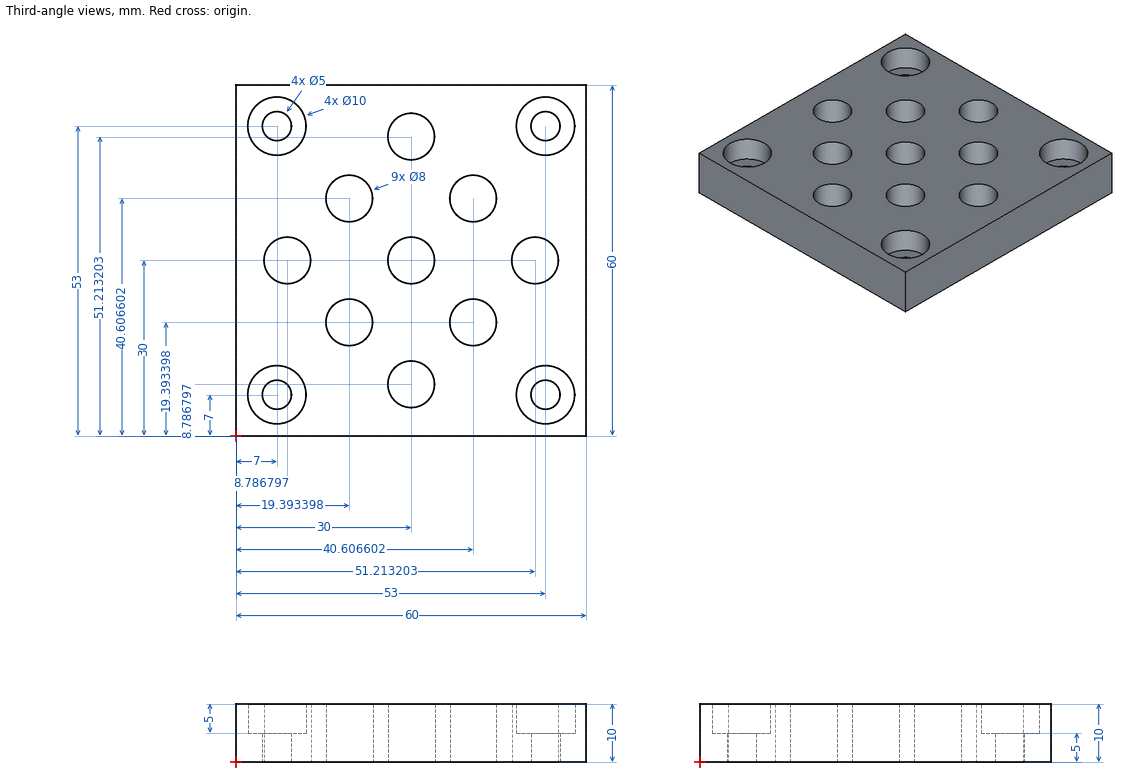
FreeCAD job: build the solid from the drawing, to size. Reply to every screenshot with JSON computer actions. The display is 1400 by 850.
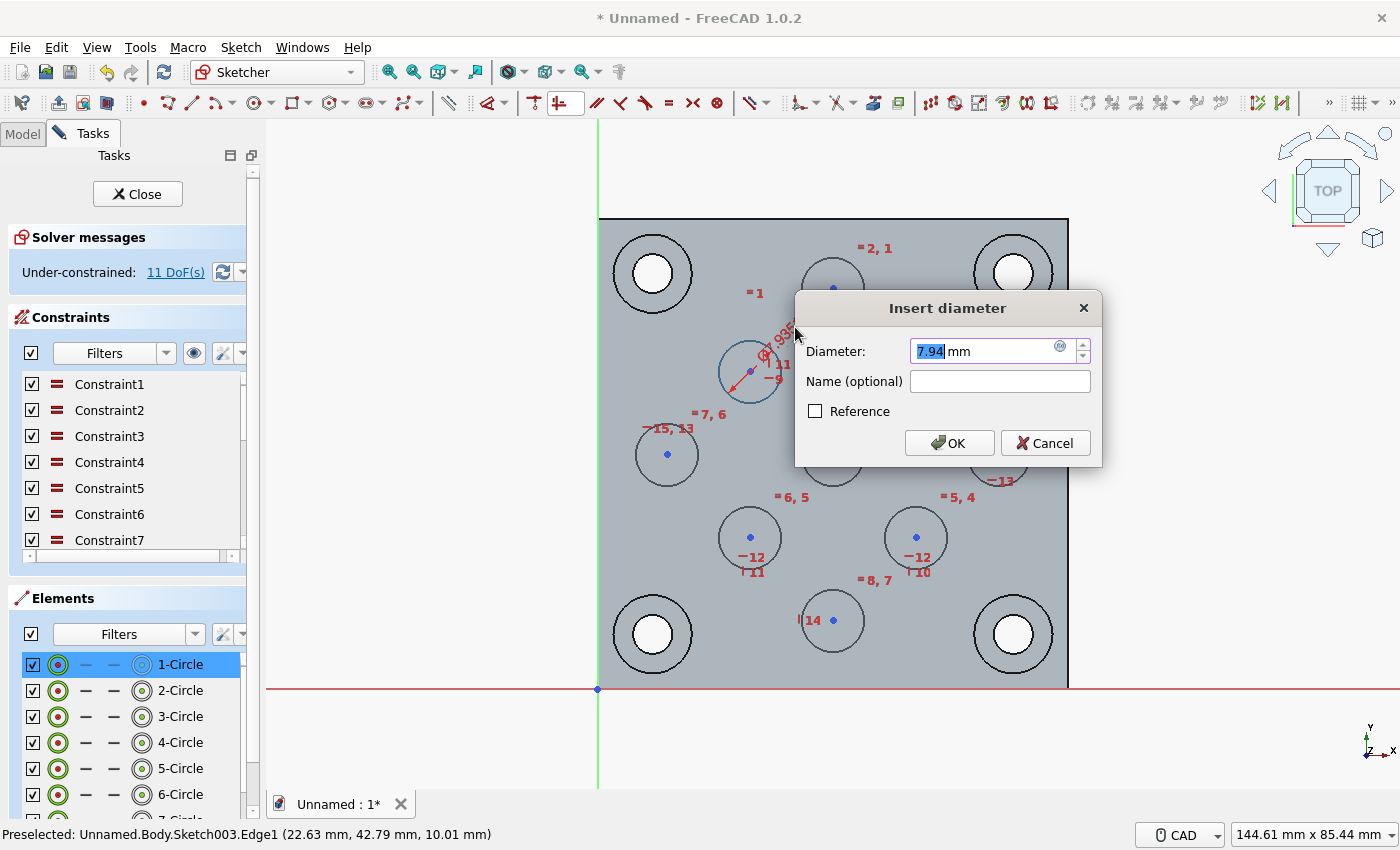
{"action": "type", "text": "8"}
{"action": "key", "text": "Return"}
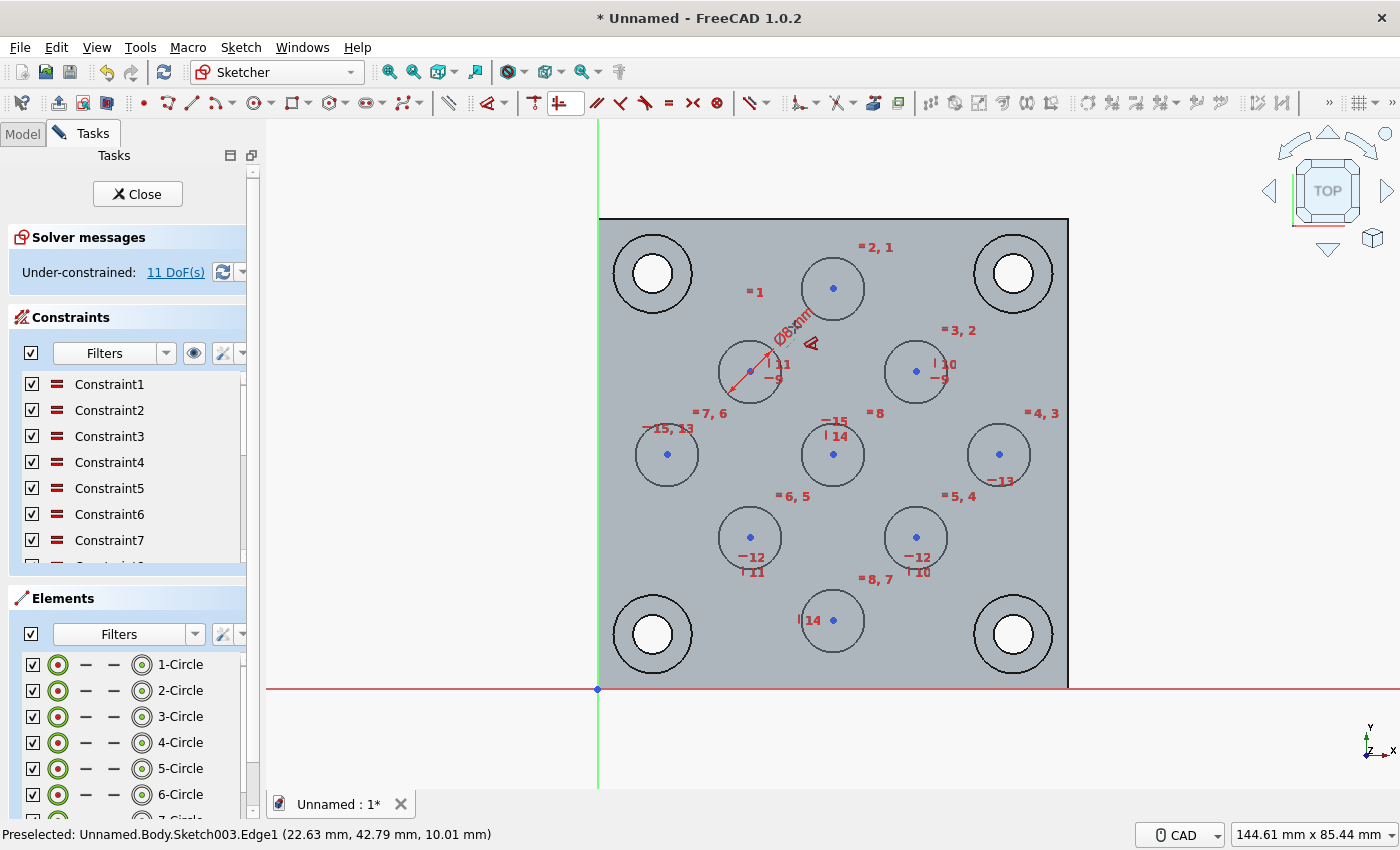
{"action": "left_click", "coordinate": [833, 289]}
{"action": "left_click", "coordinate": [715, 723]}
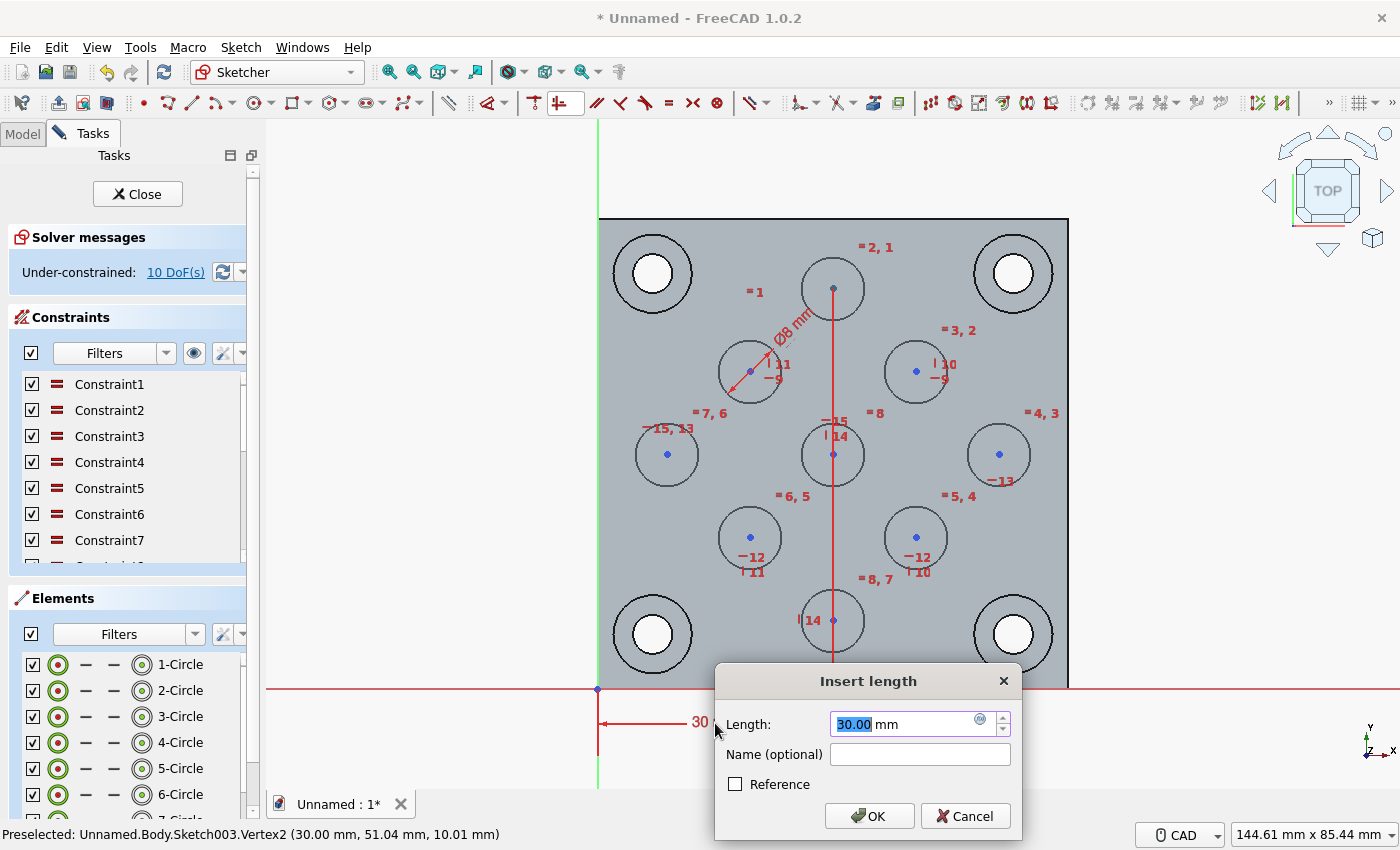
{"action": "type", "text": "30"}
{"action": "key", "text": "Return"}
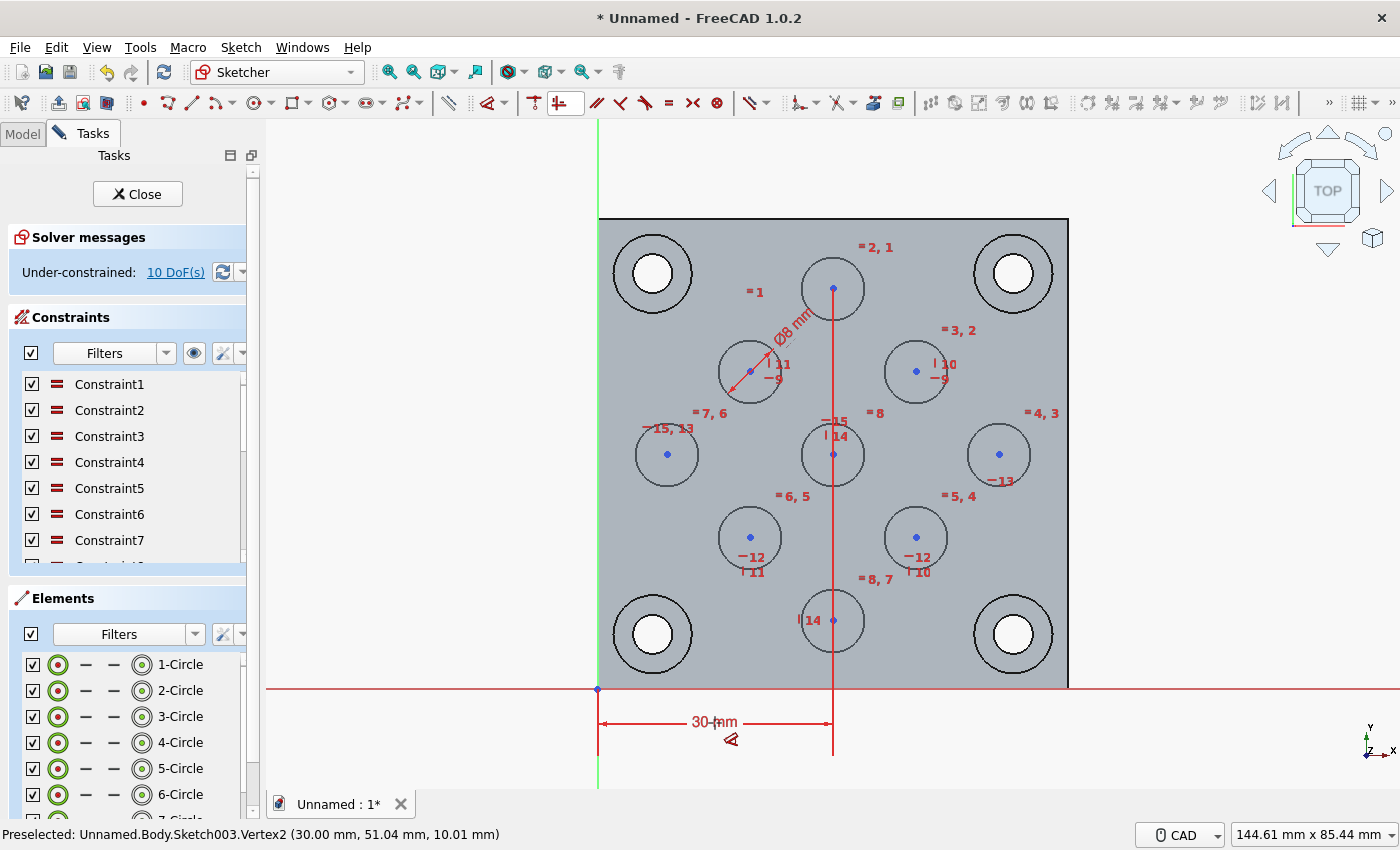
{"action": "left_click", "coordinate": [999, 455]}
{"action": "left_click", "coordinate": [564, 572]}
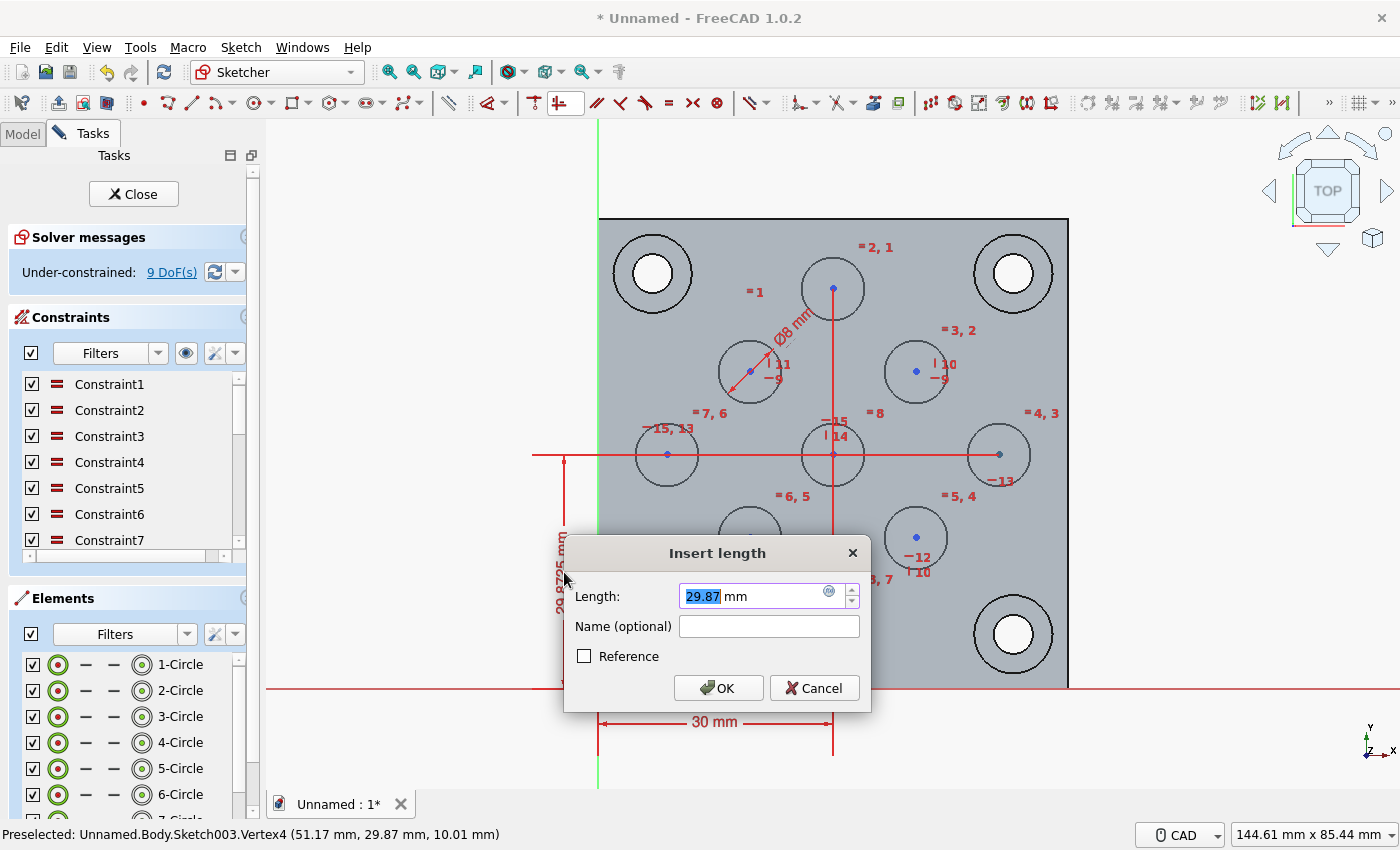
{"action": "type", "text": "30"}
{"action": "key", "text": "Return"}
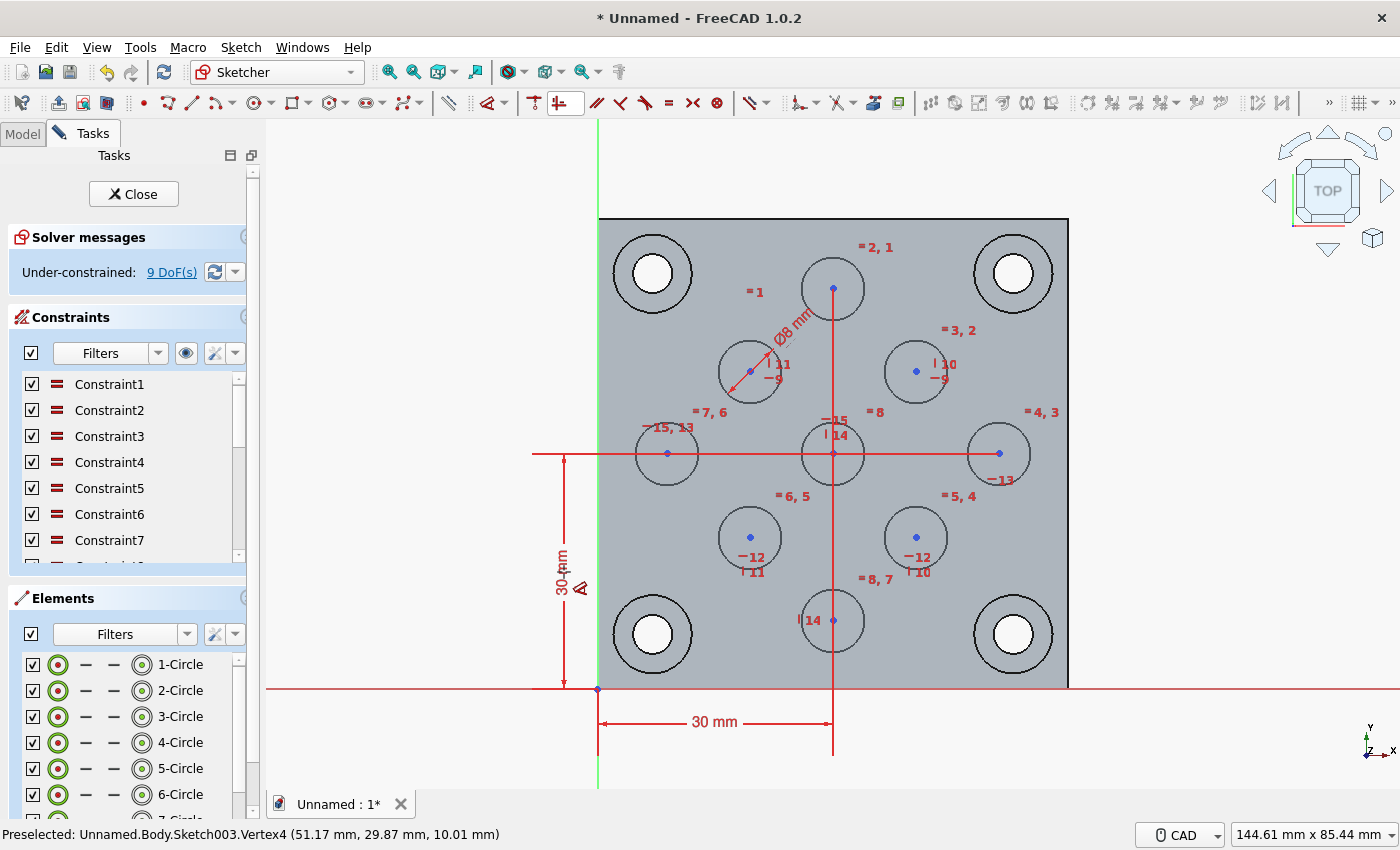
{"action": "left_click", "coordinate": [833, 621]}
{"action": "left_click", "coordinate": [633, 723]}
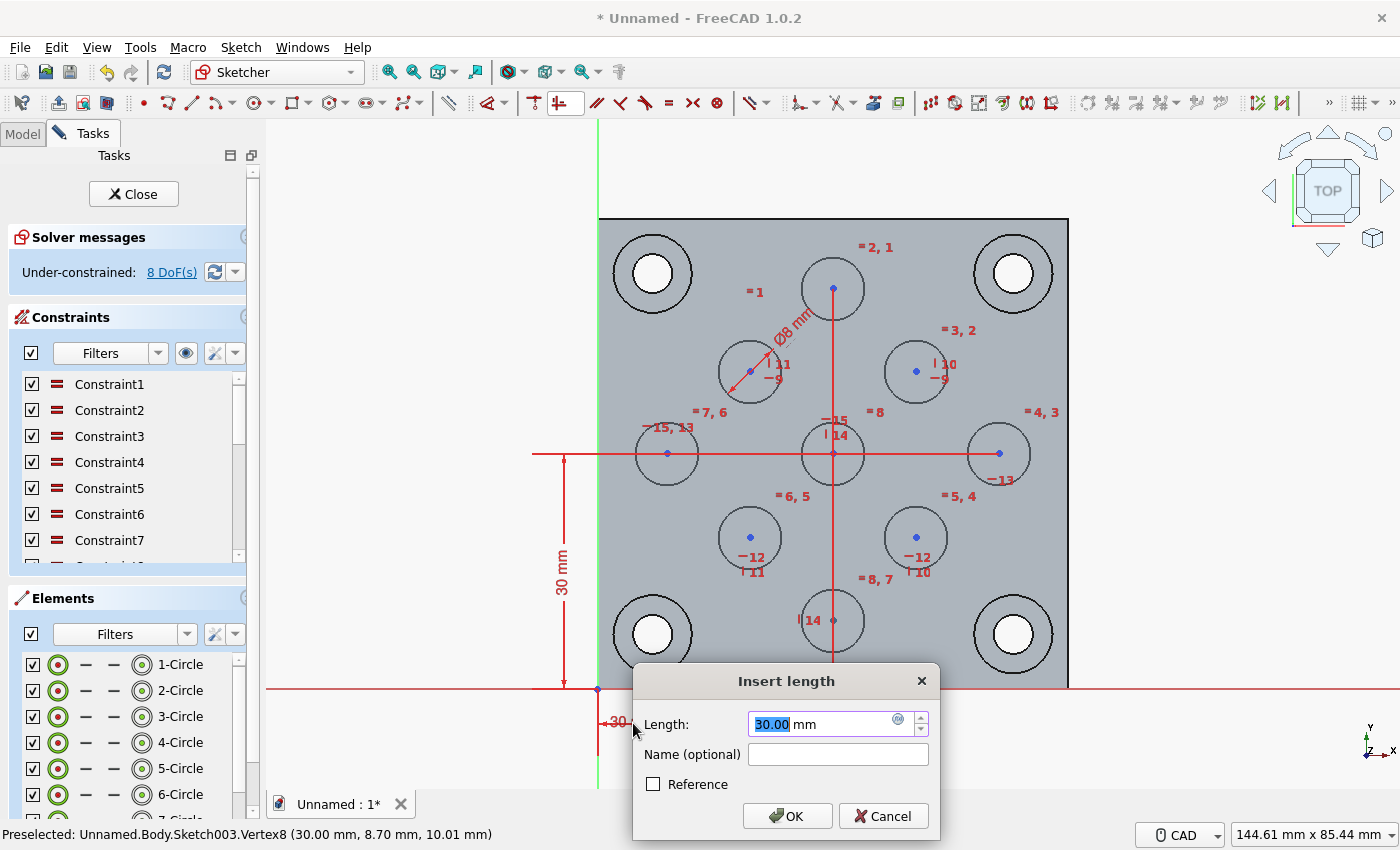
{"action": "type", "text": "30"}
{"action": "key", "text": "Return"}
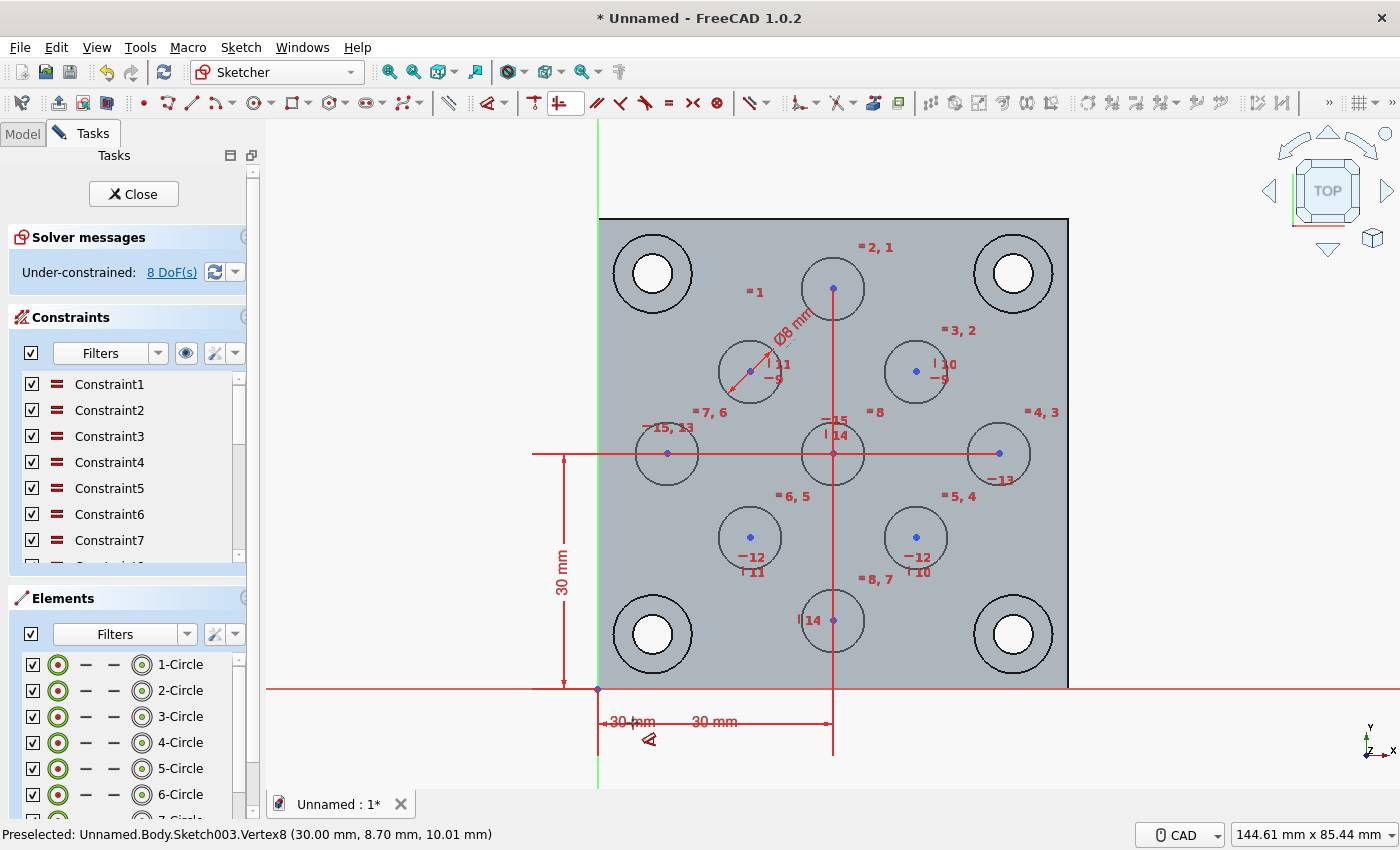
{"action": "left_click", "coordinate": [667, 454]}
{"action": "left_click", "coordinate": [632, 420]}